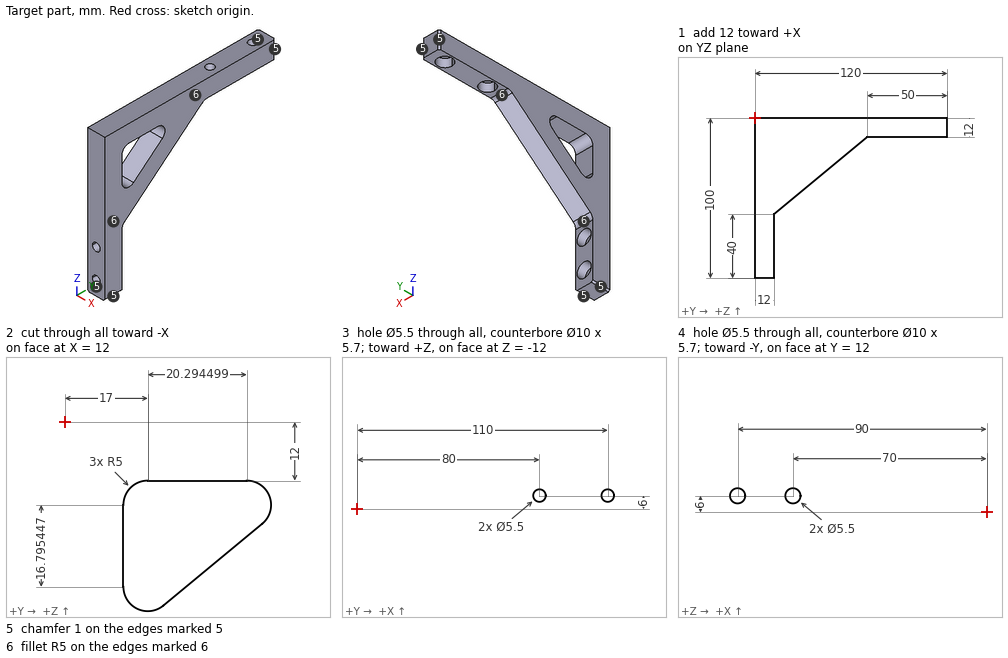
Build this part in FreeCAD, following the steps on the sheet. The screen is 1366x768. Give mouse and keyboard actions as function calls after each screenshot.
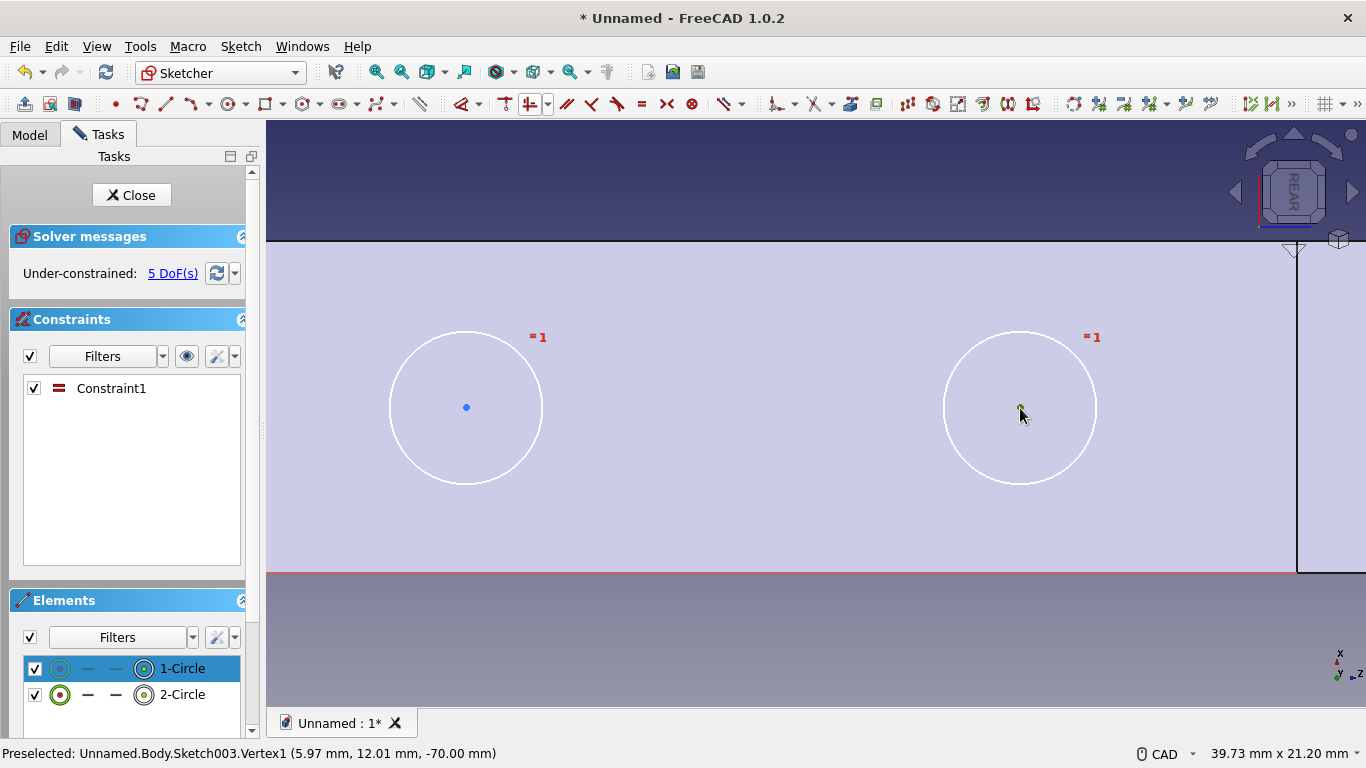
click(466, 408)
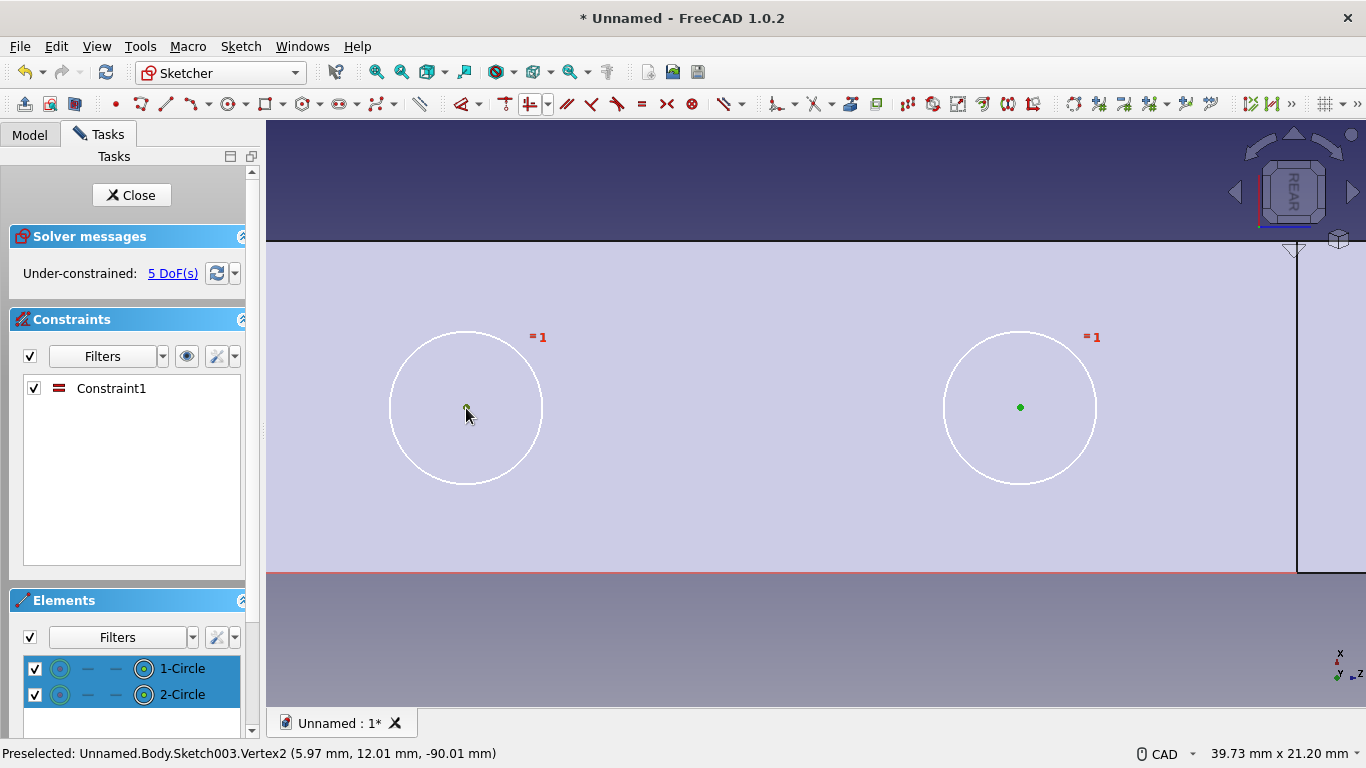
click(548, 104)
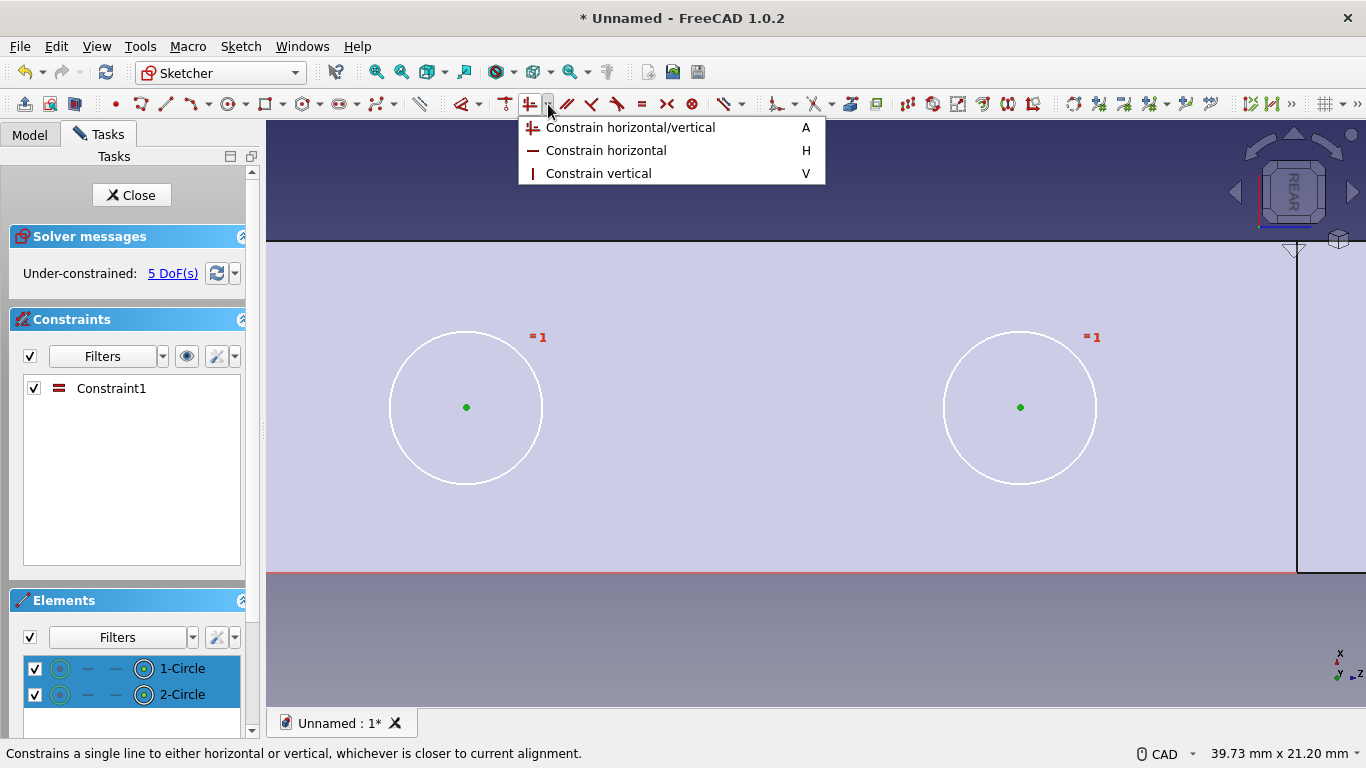
click(672, 150)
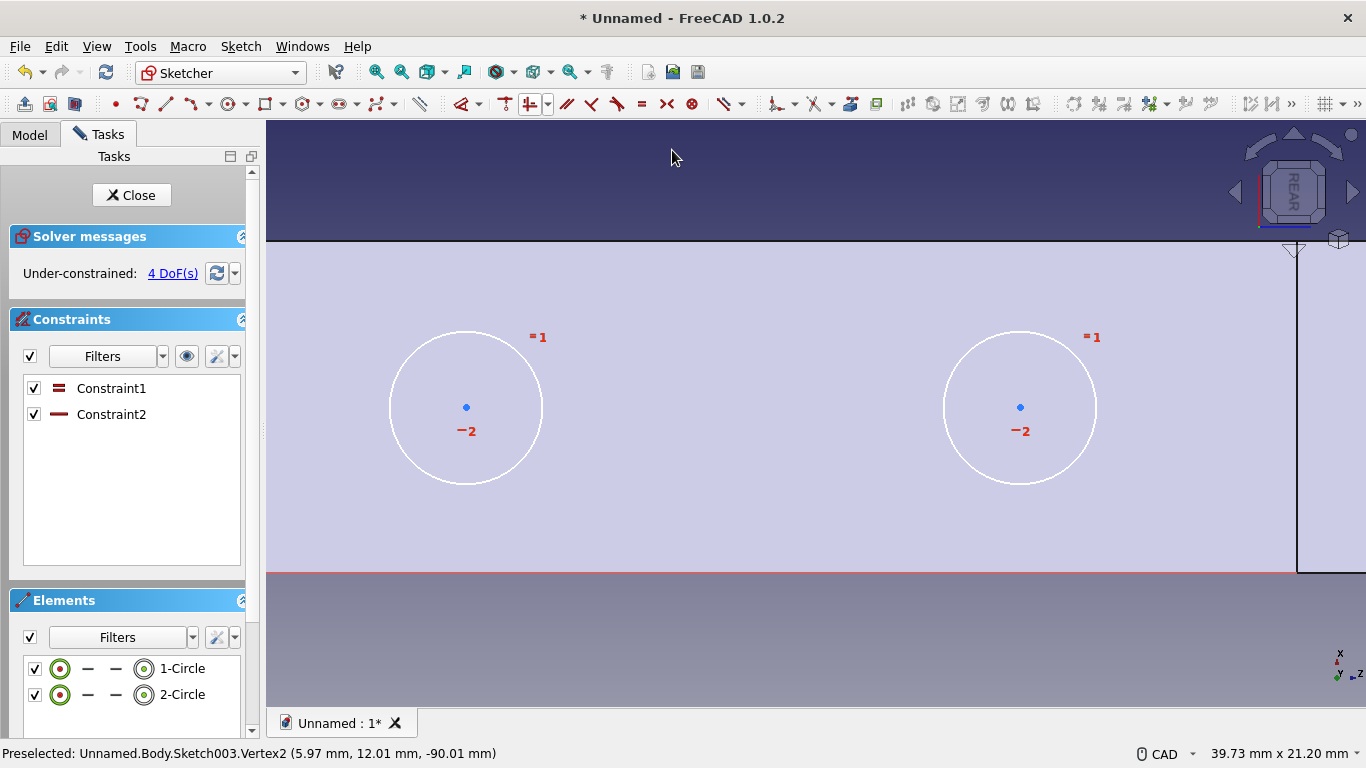
click(460, 104)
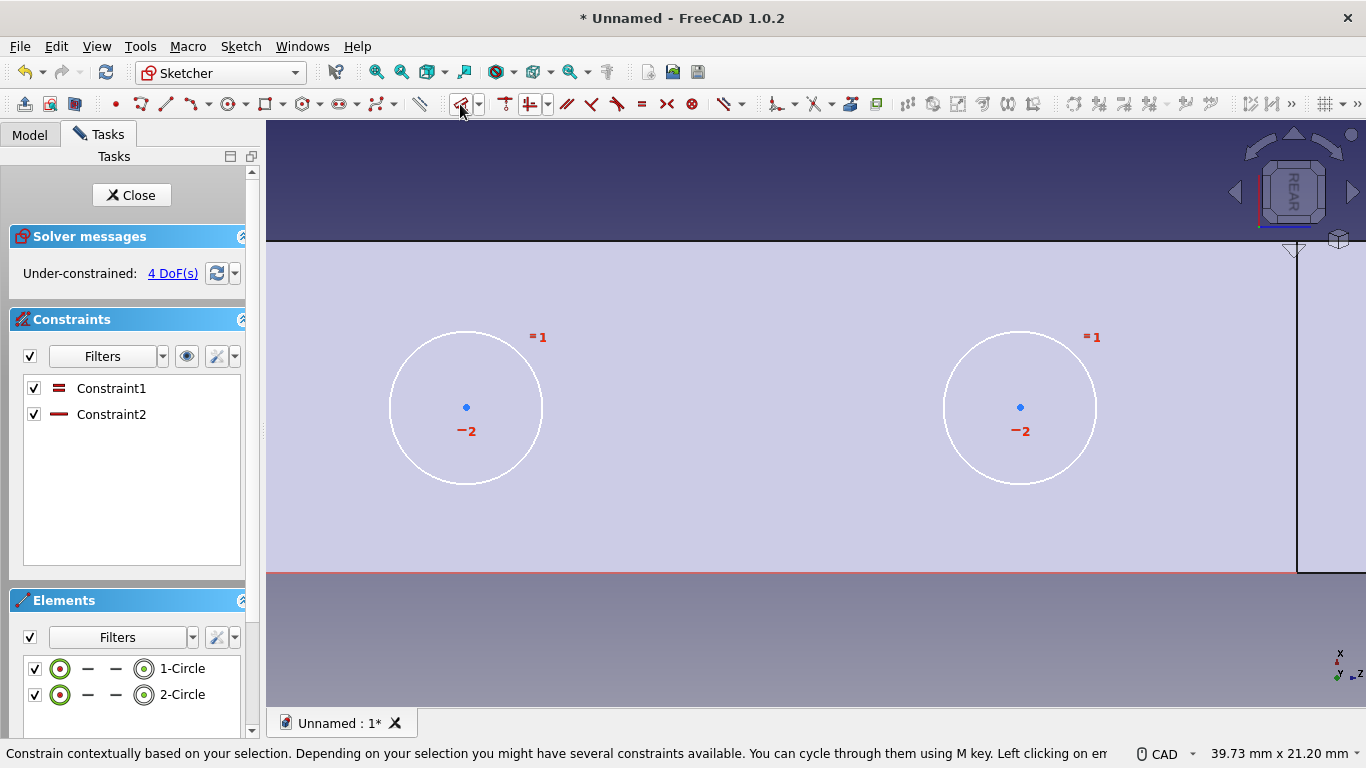
click(1074, 354)
click(1097, 331)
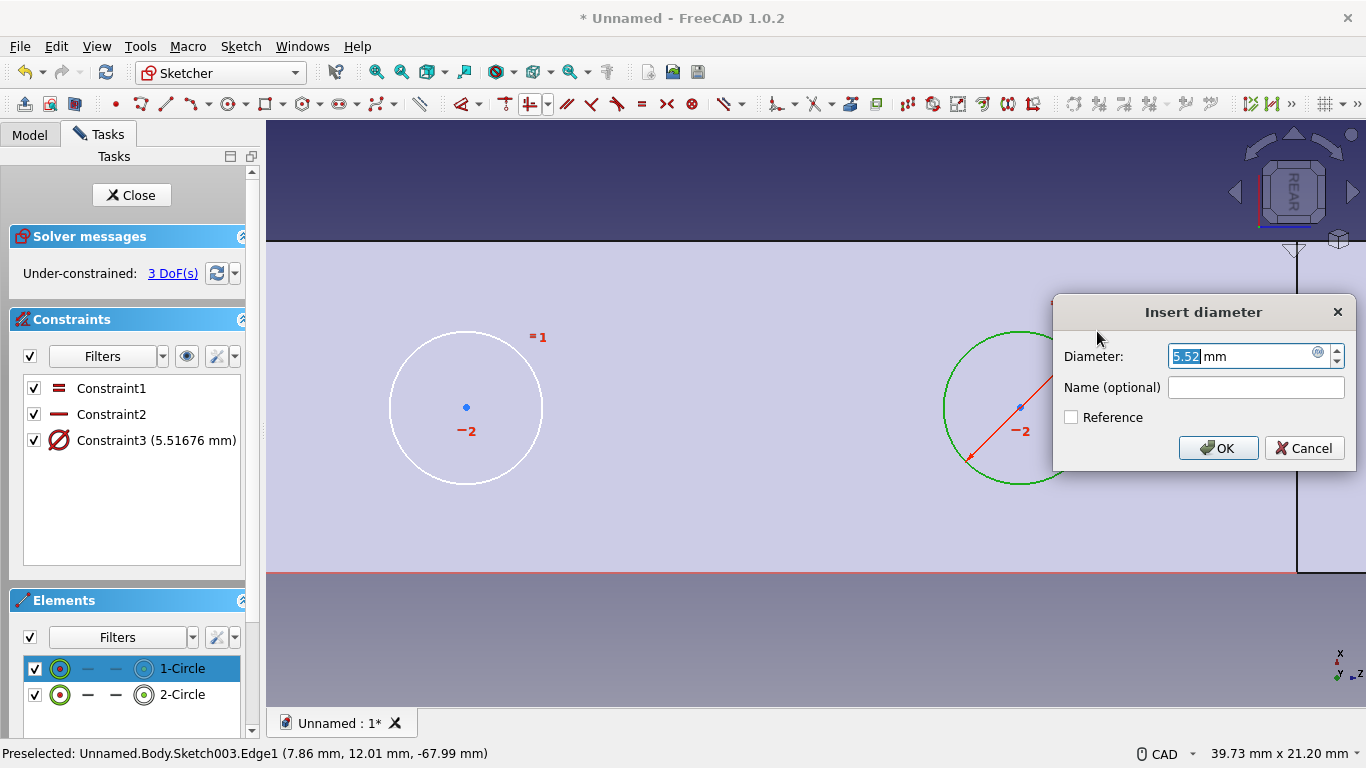
text(5.5)
key(Return)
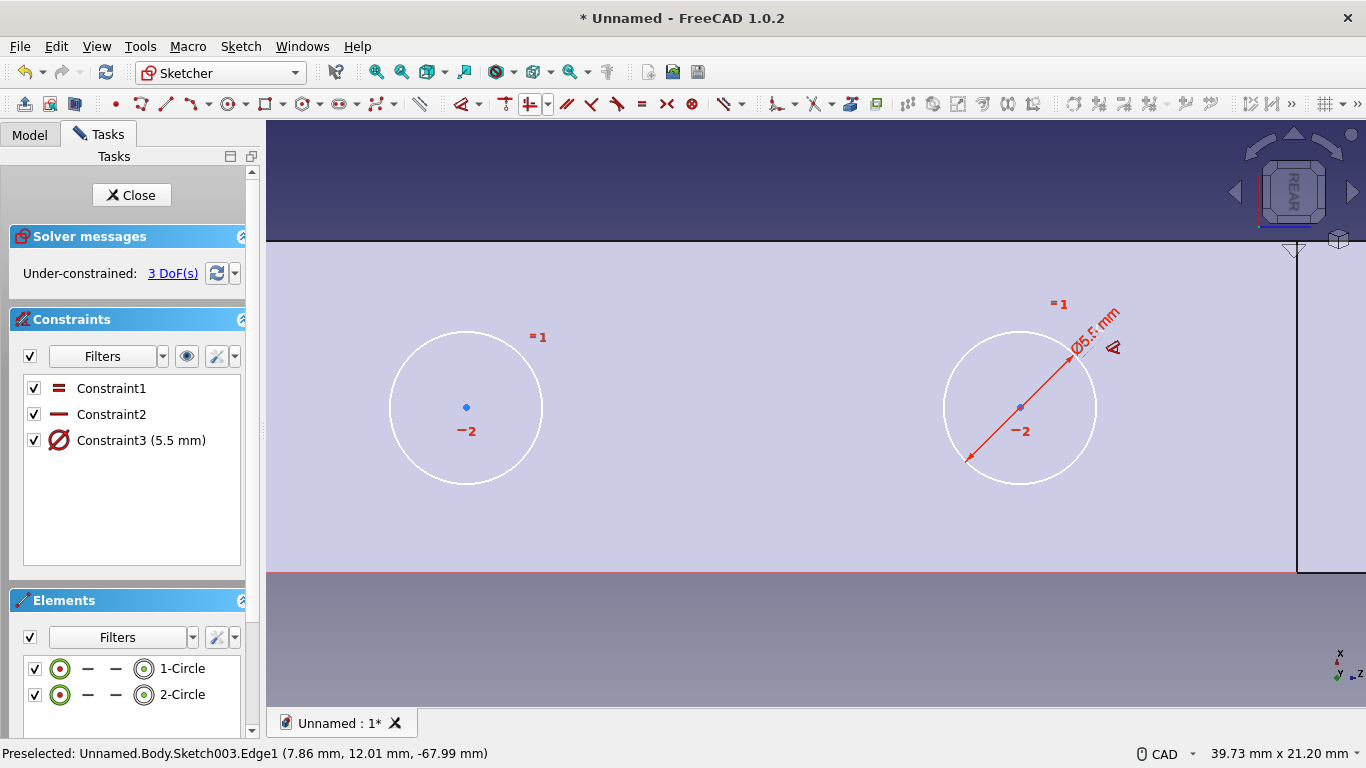
click(1020, 408)
click(986, 491)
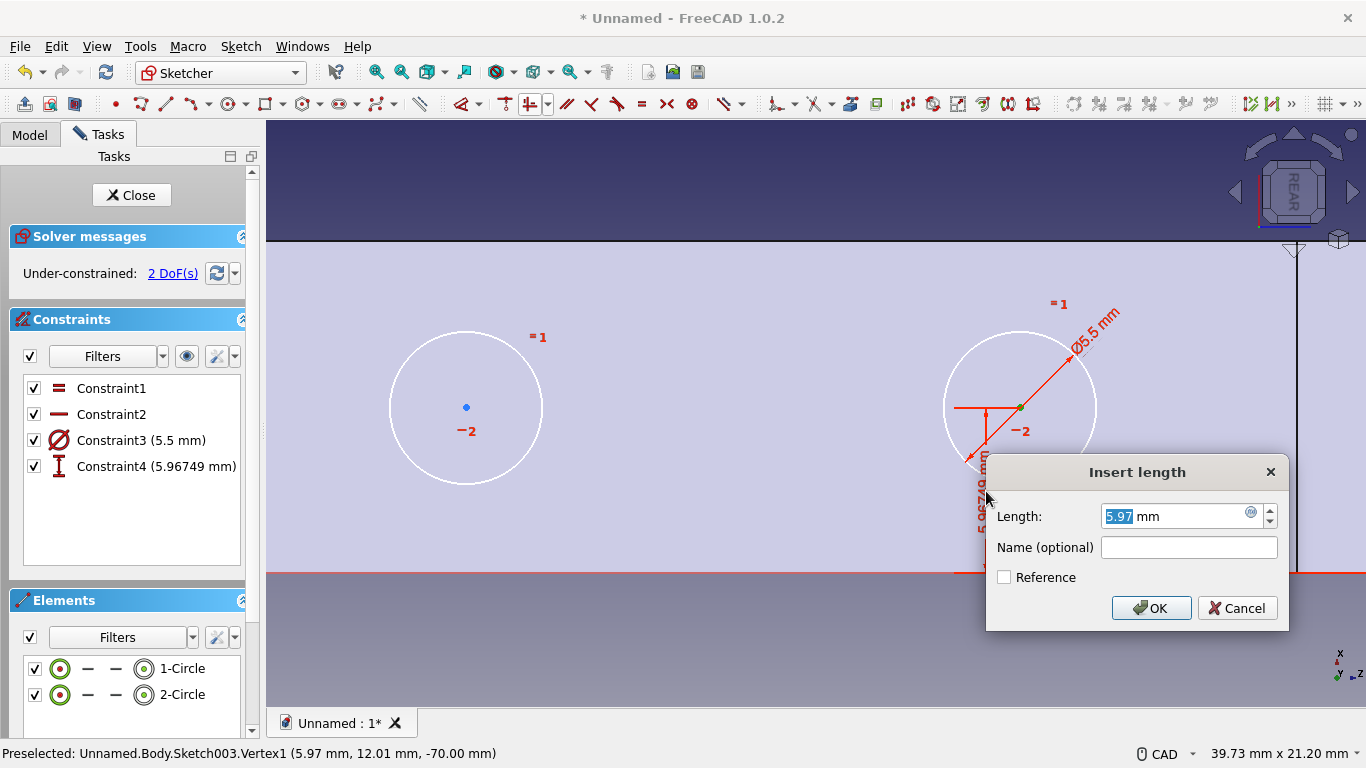
text(6)
key(Return)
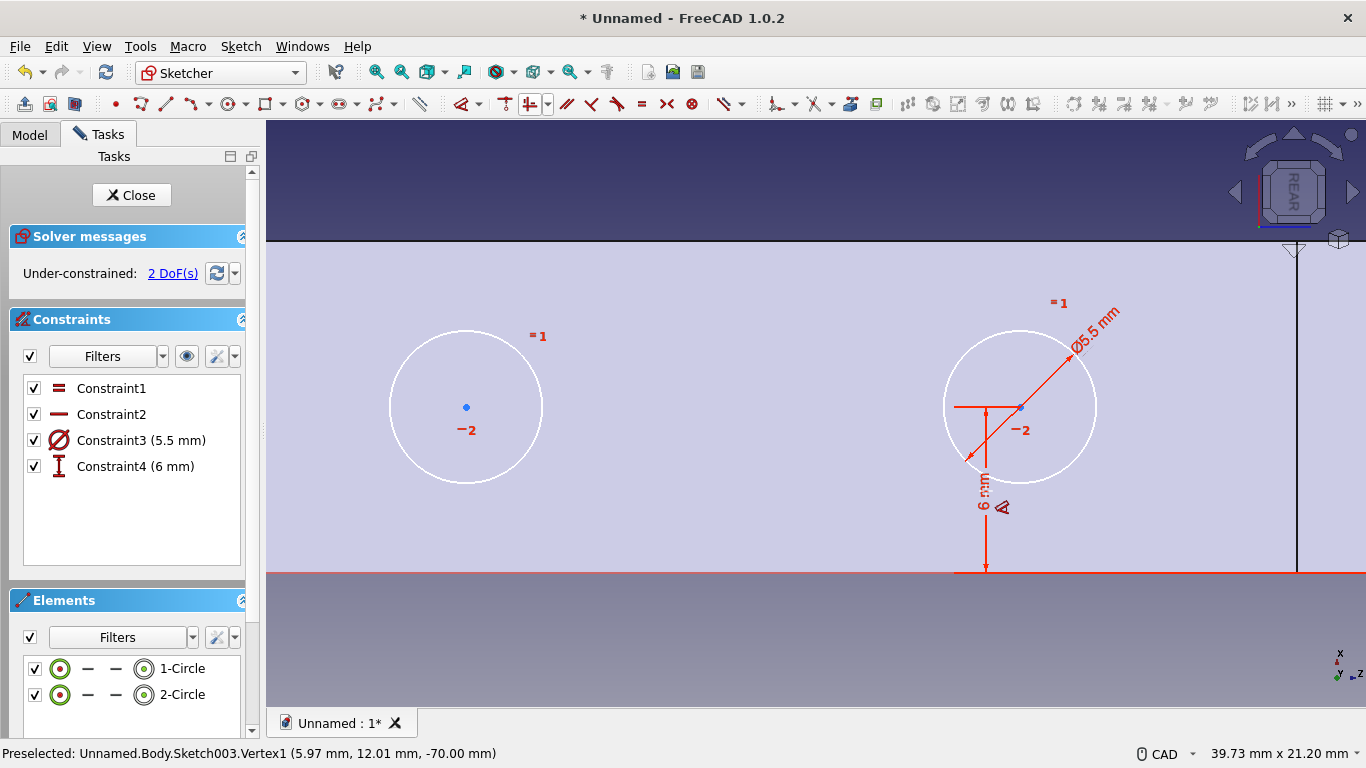
click(1020, 407)
click(1111, 607)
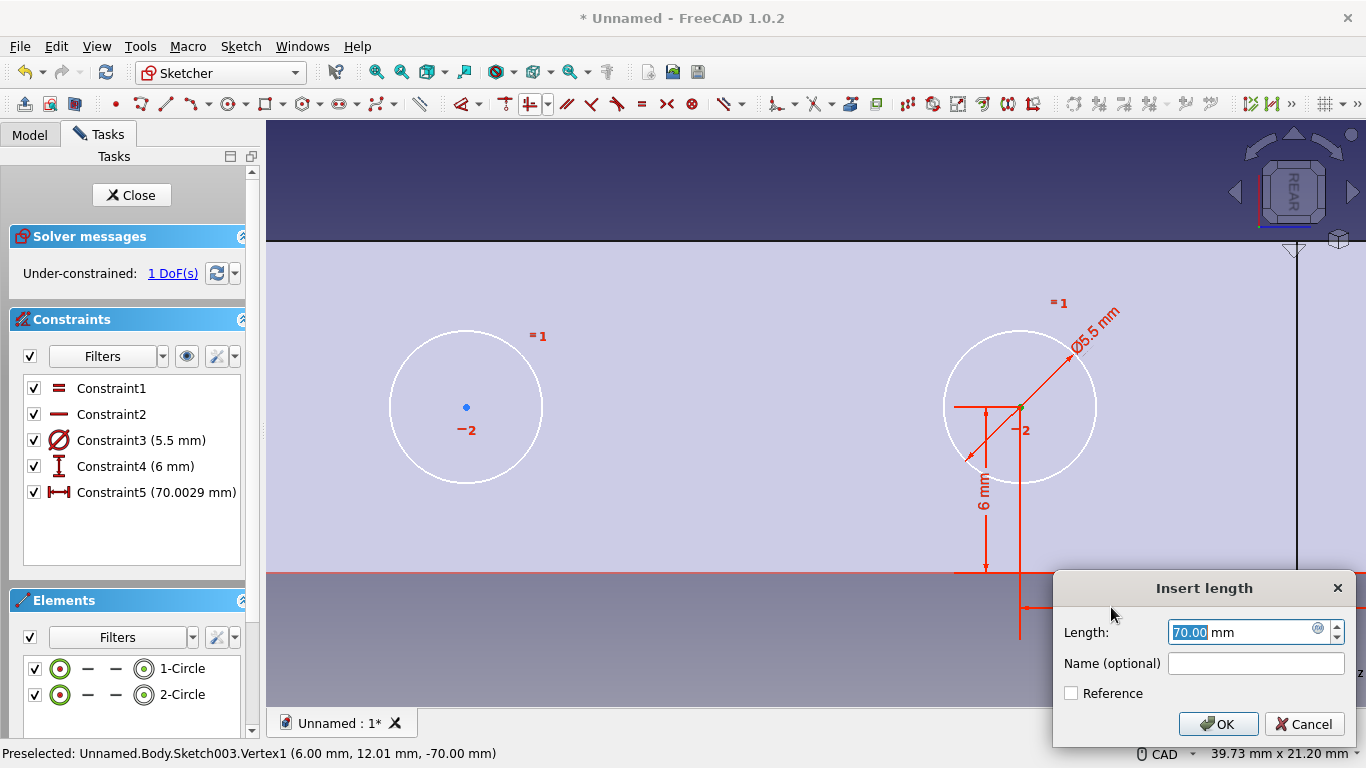
text(70)
key(Return)